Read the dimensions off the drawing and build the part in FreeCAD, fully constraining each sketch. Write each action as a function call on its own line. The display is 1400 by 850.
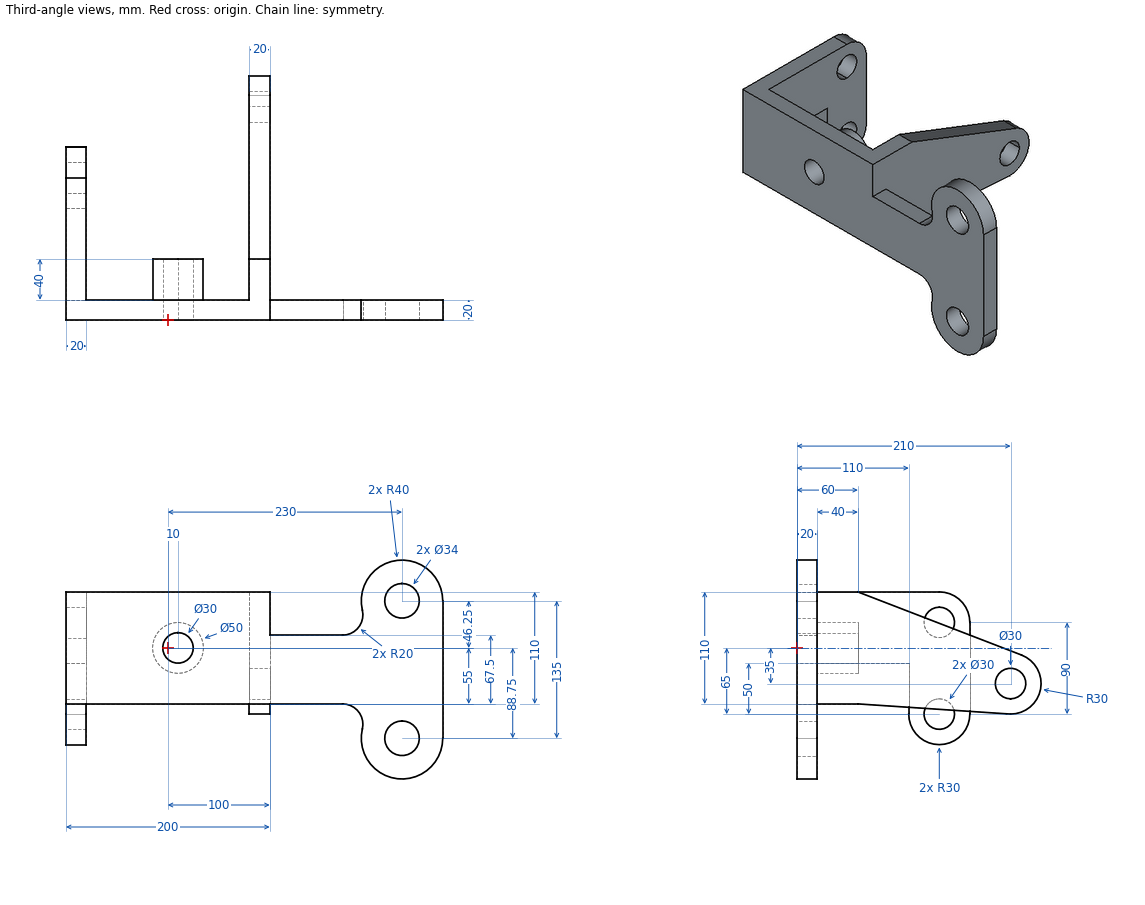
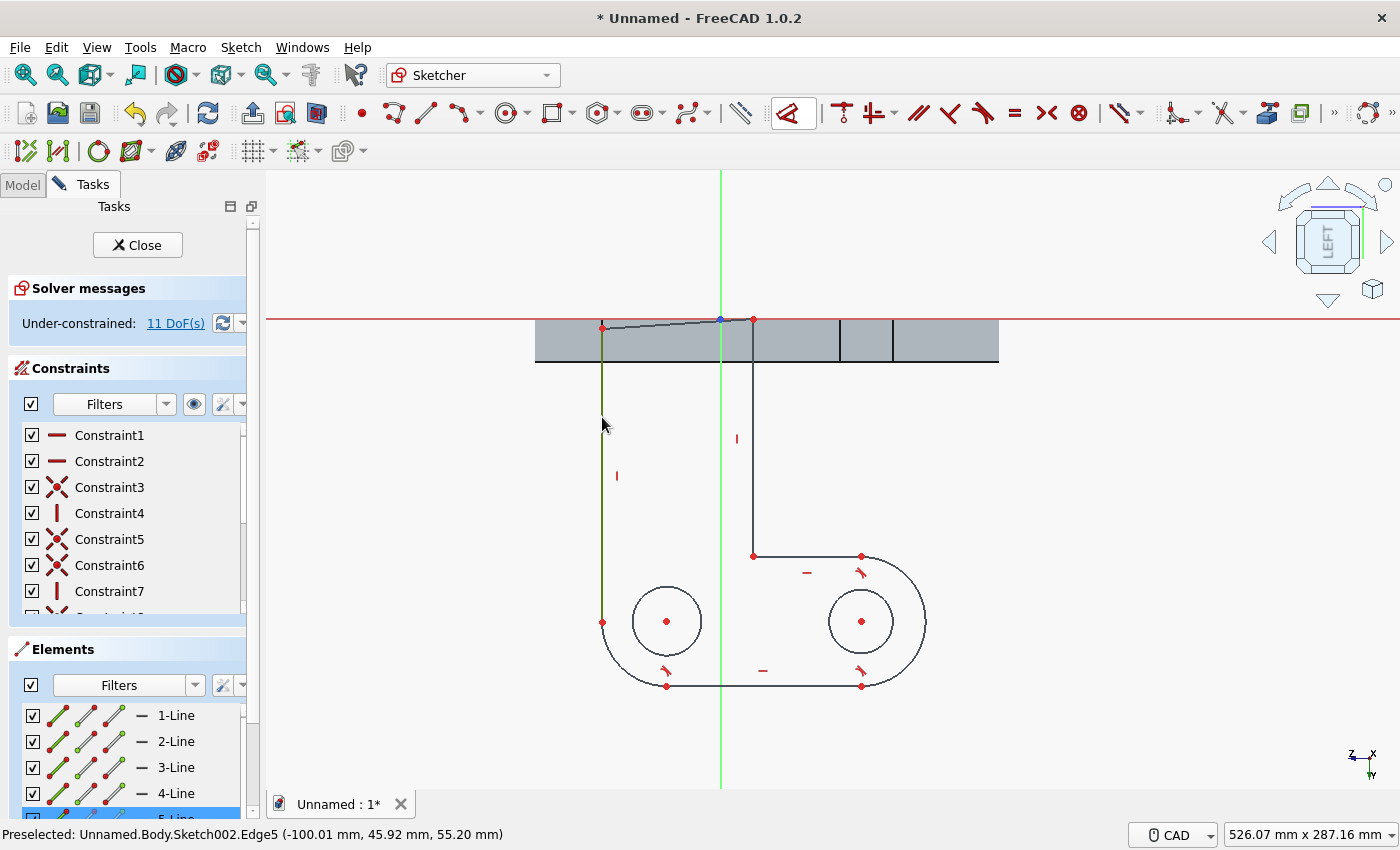
click(609, 651)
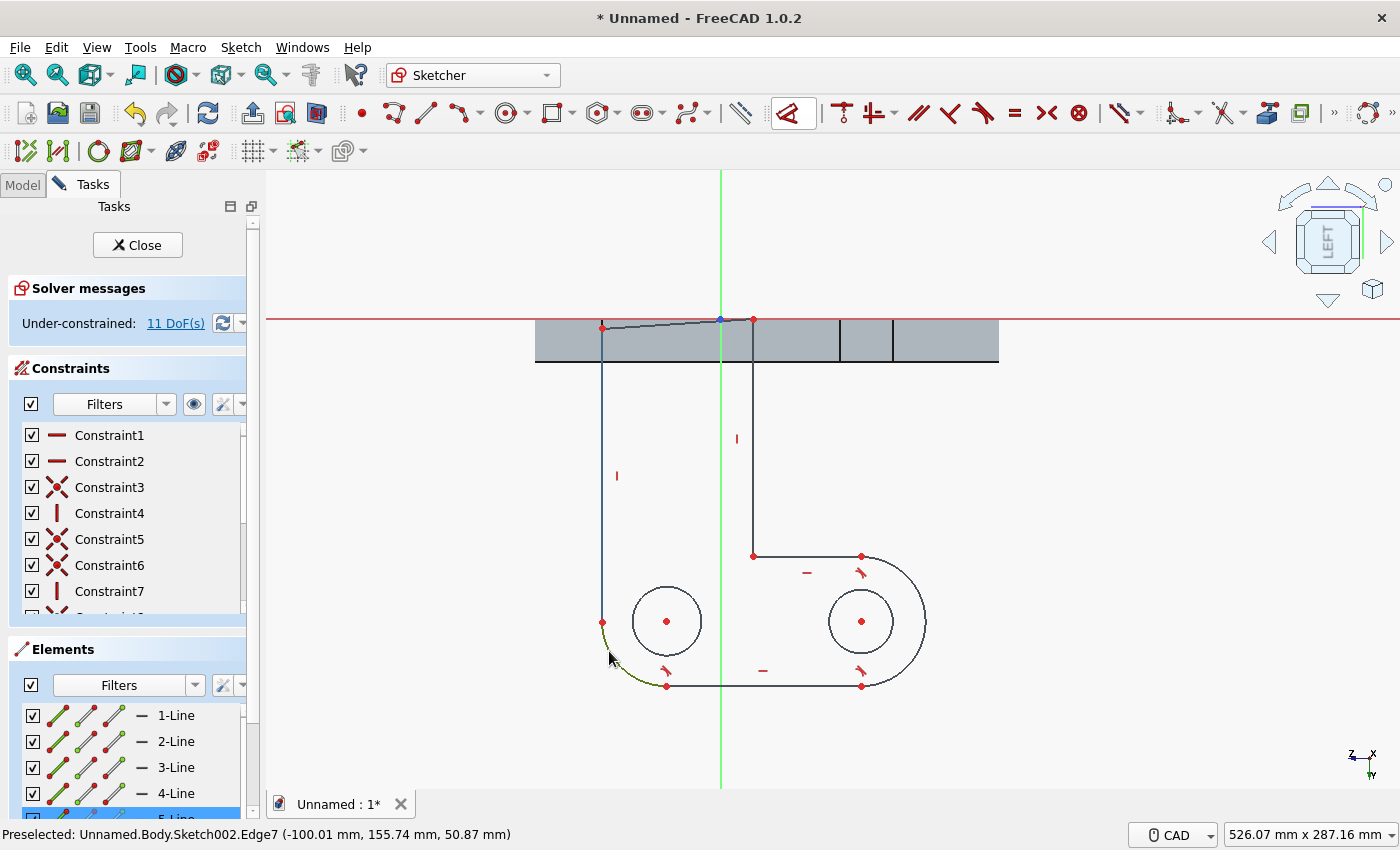
click(984, 114)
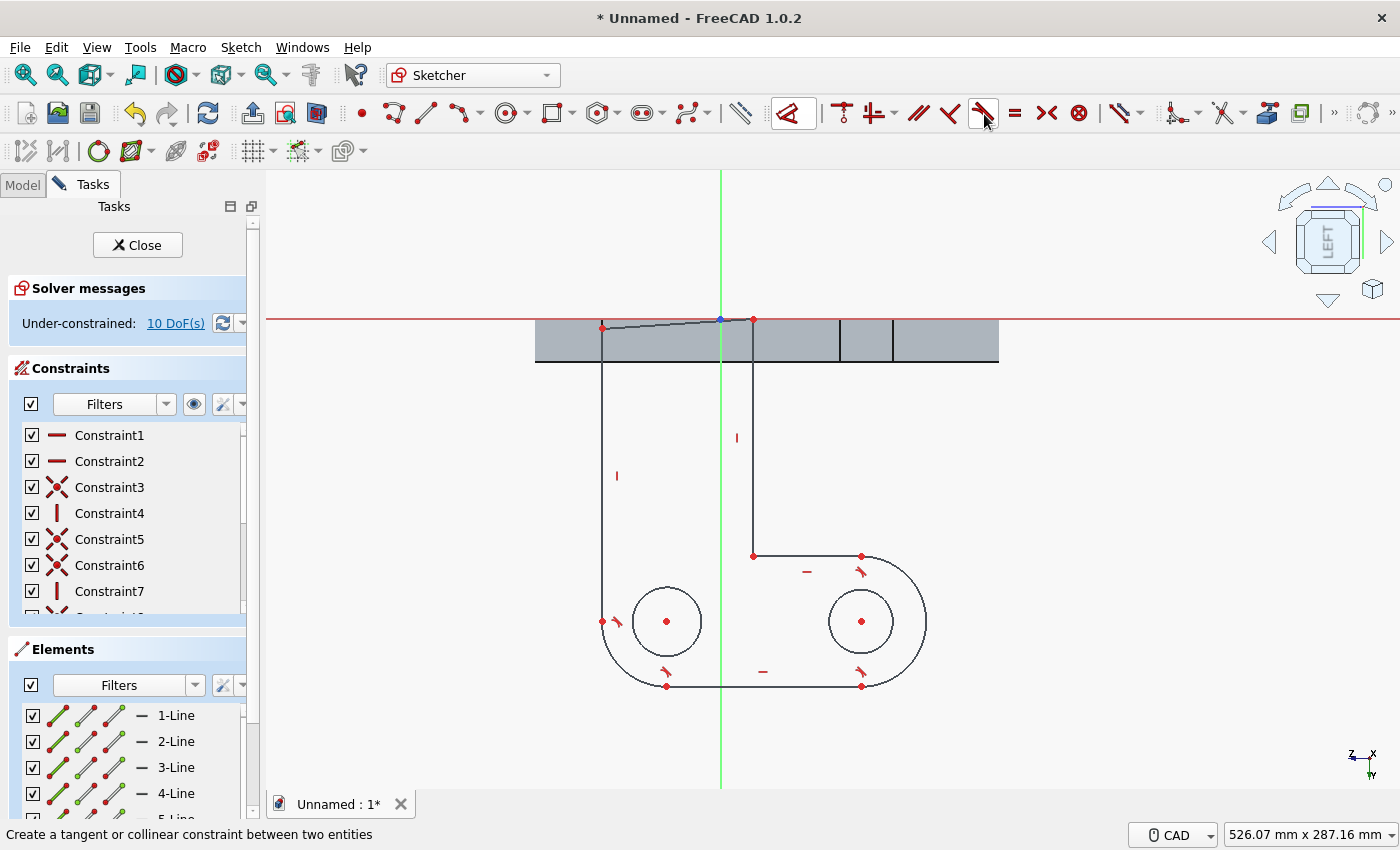
click(708, 322)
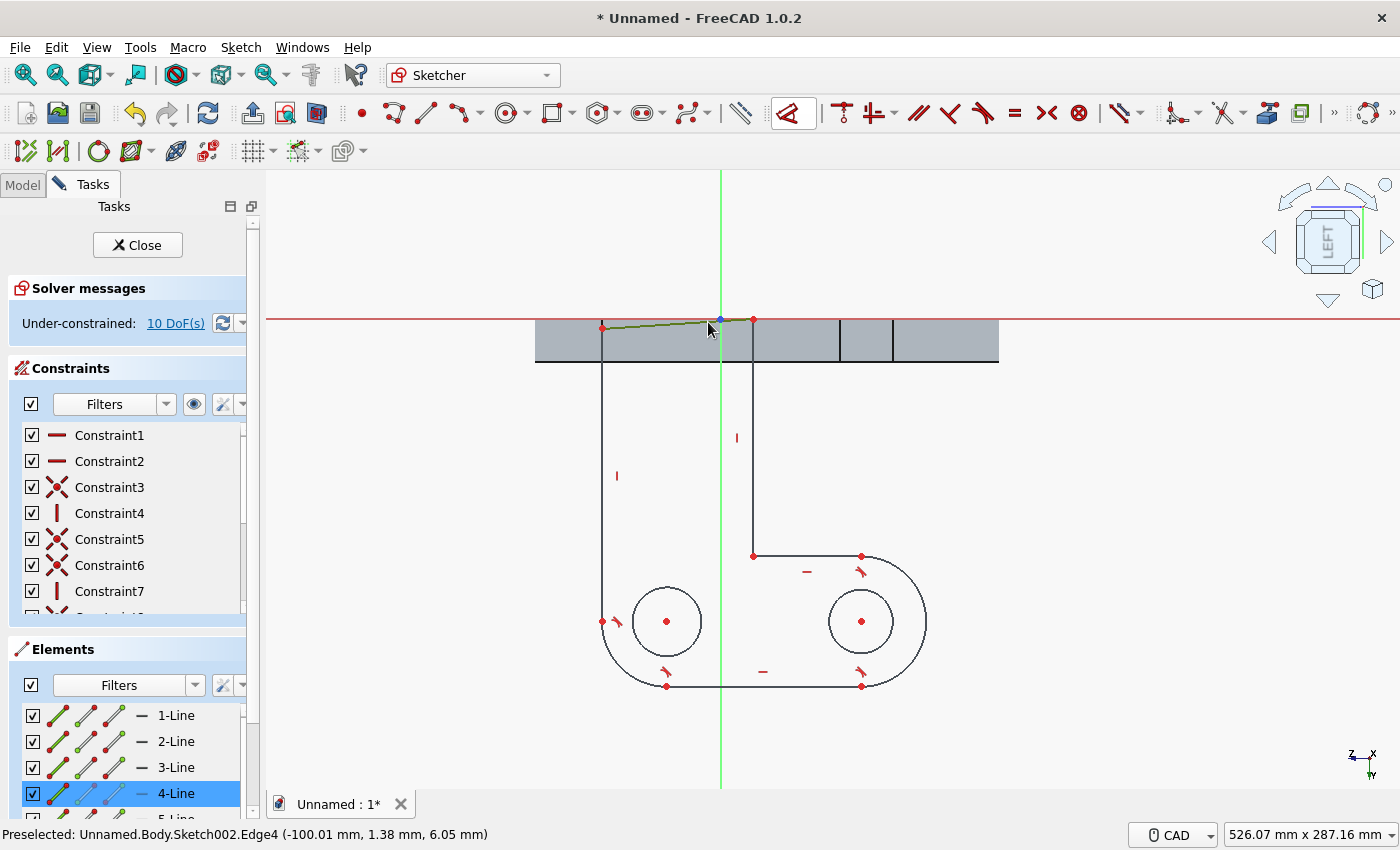
key(h)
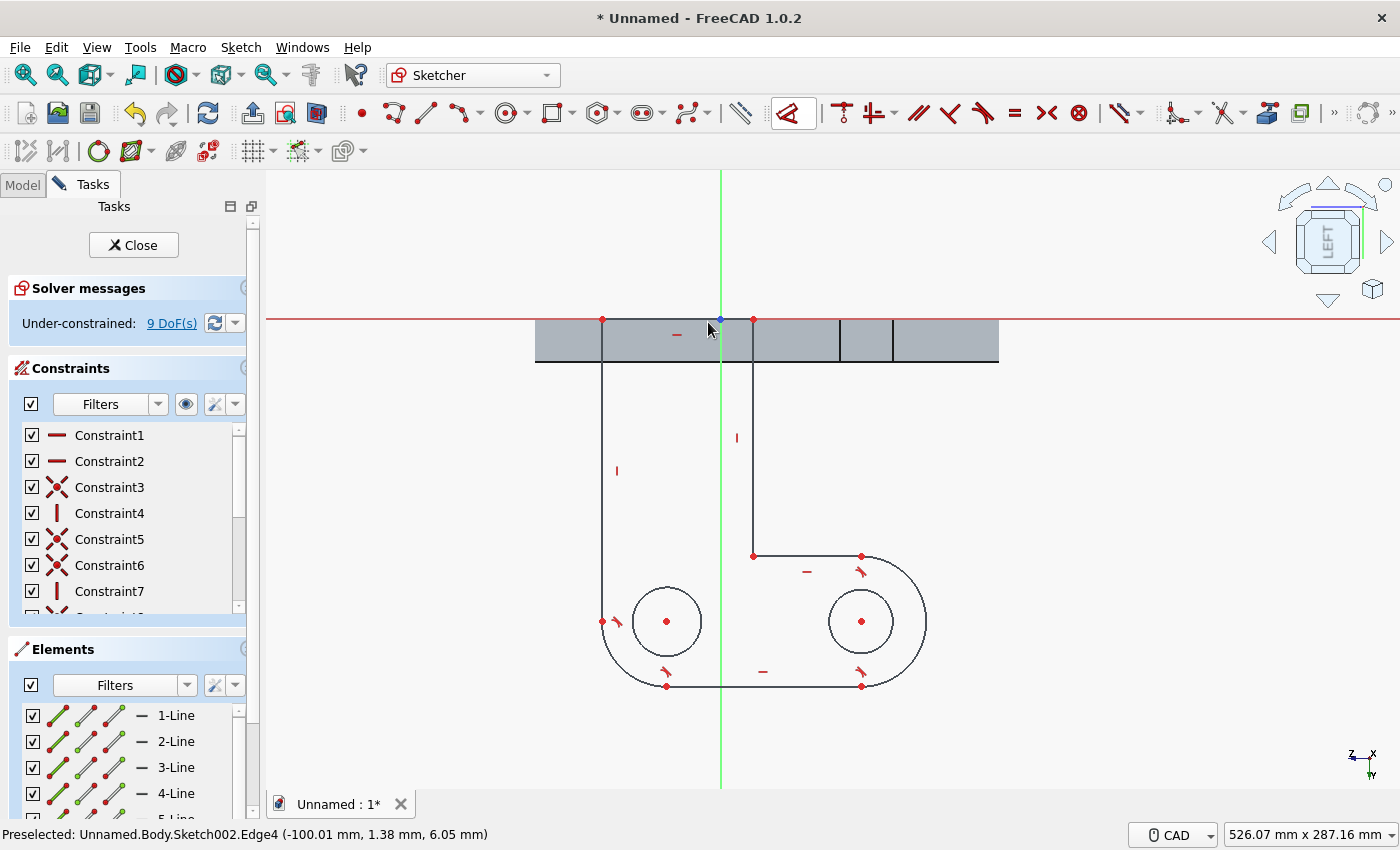
click(914, 660)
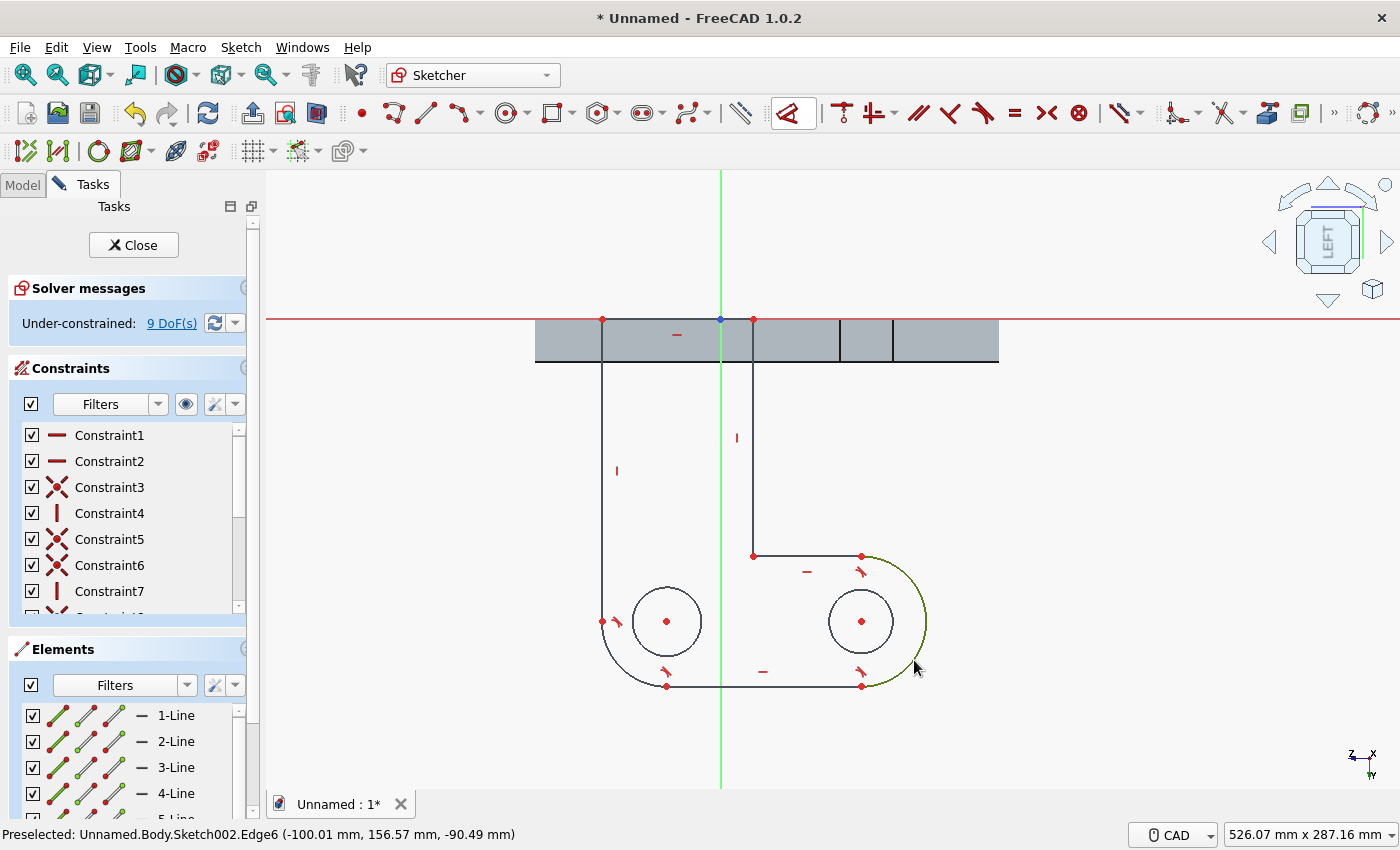
click(609, 651)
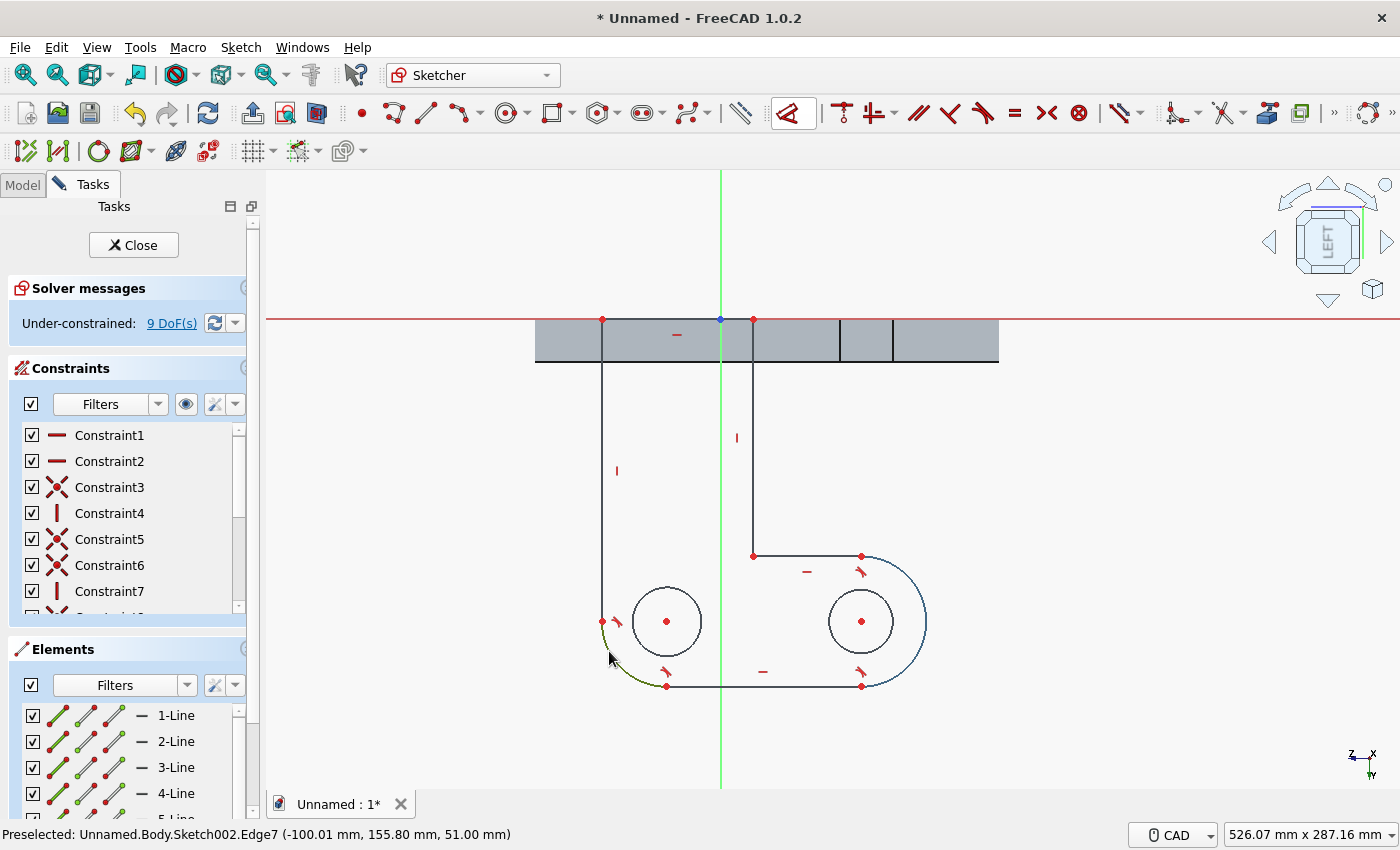
click(1016, 114)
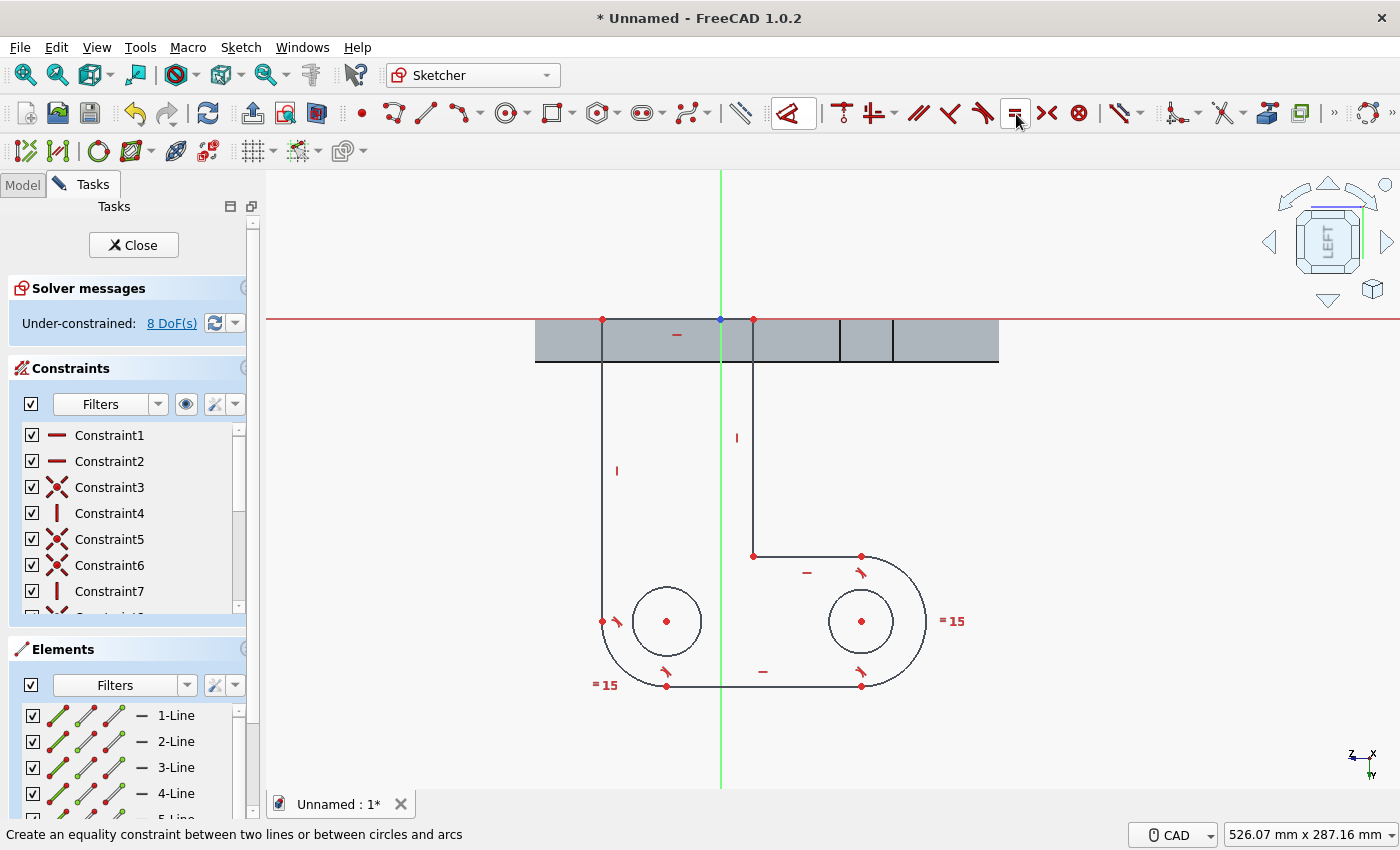
click(883, 599)